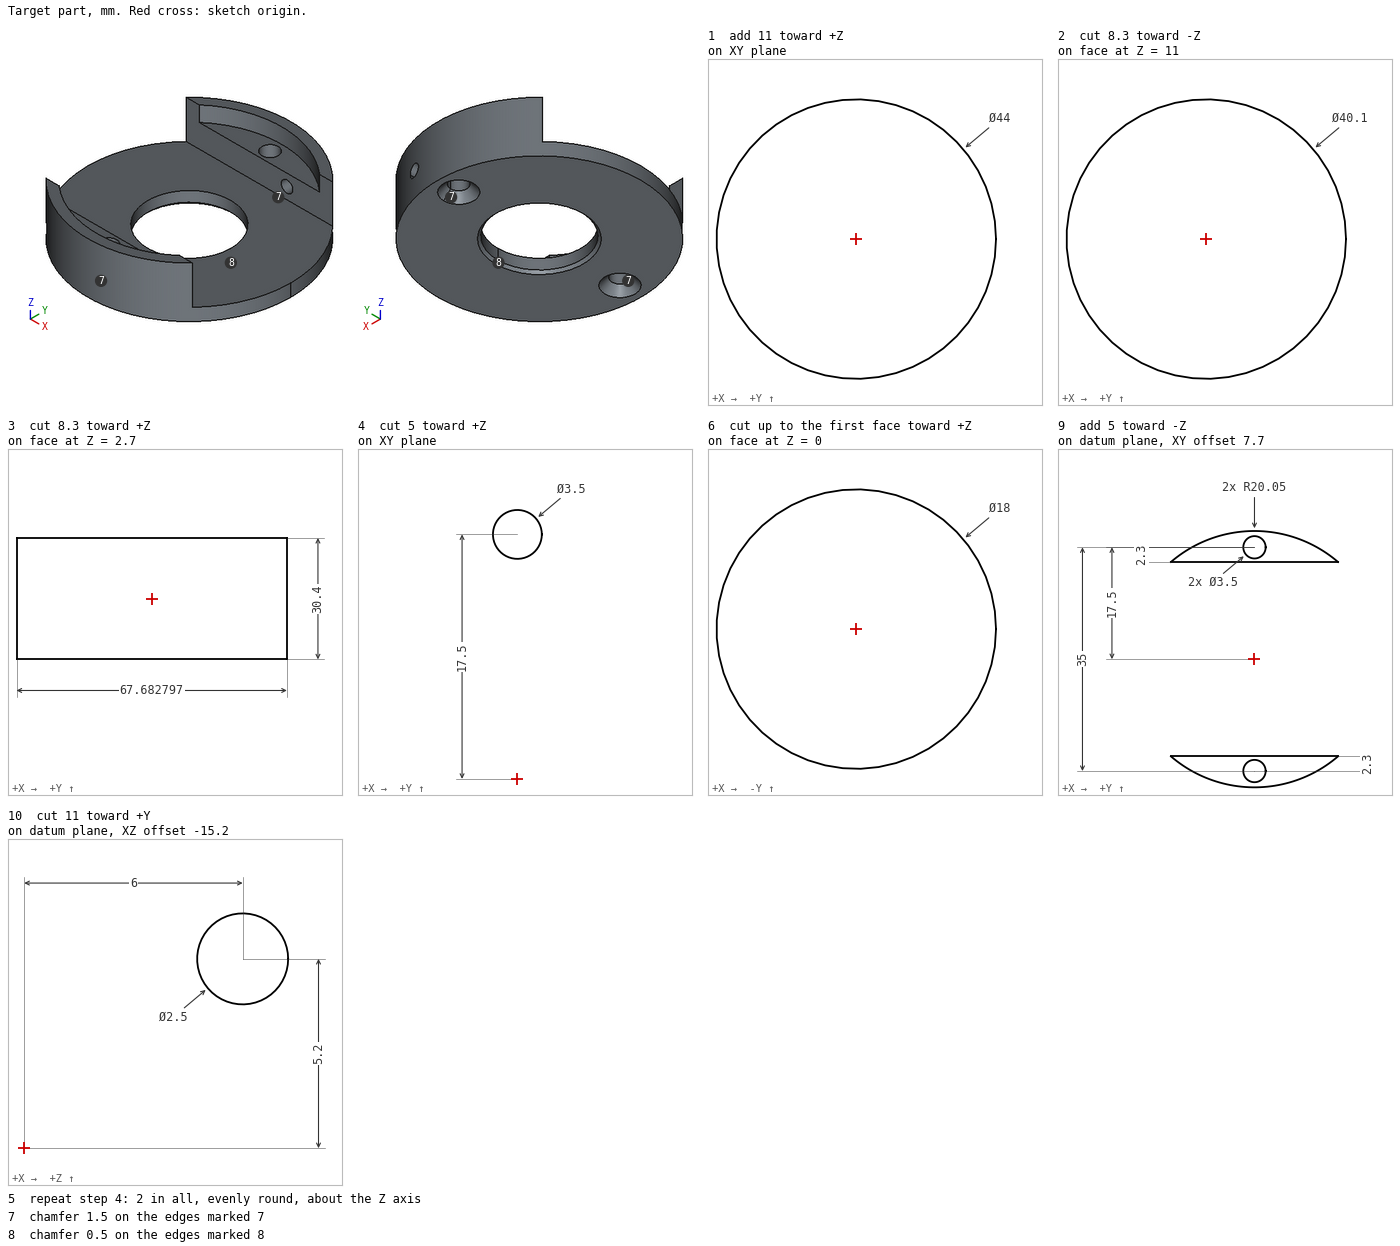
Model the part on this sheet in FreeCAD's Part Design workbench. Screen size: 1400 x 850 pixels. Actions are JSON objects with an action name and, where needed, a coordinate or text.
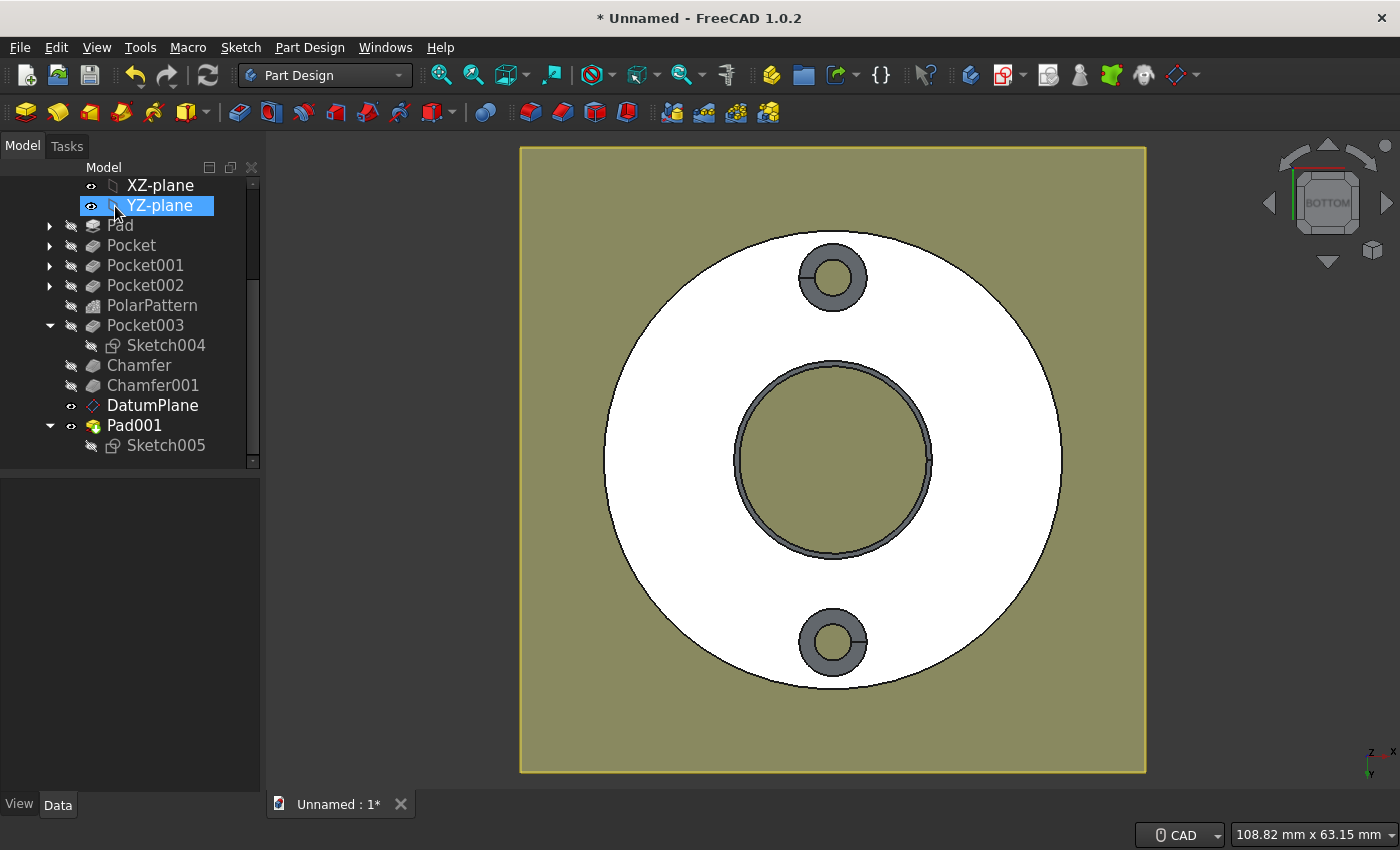
{"action": "left_click", "coordinate": [116, 406]}
{"action": "key", "text": "space"}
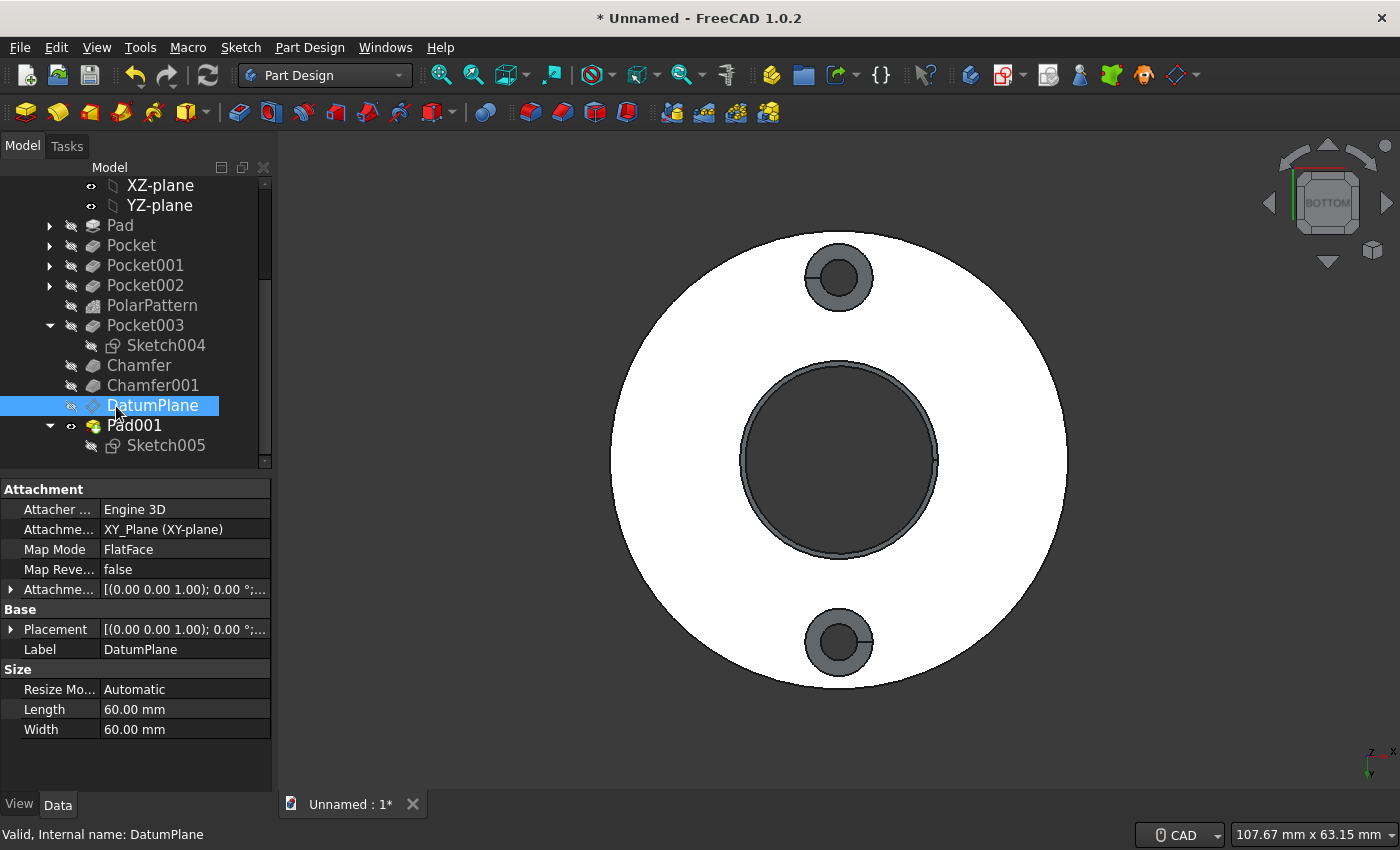
{"action": "scroll", "coordinate": [160, 321], "scroll_direction": "down", "scroll_amount": 3}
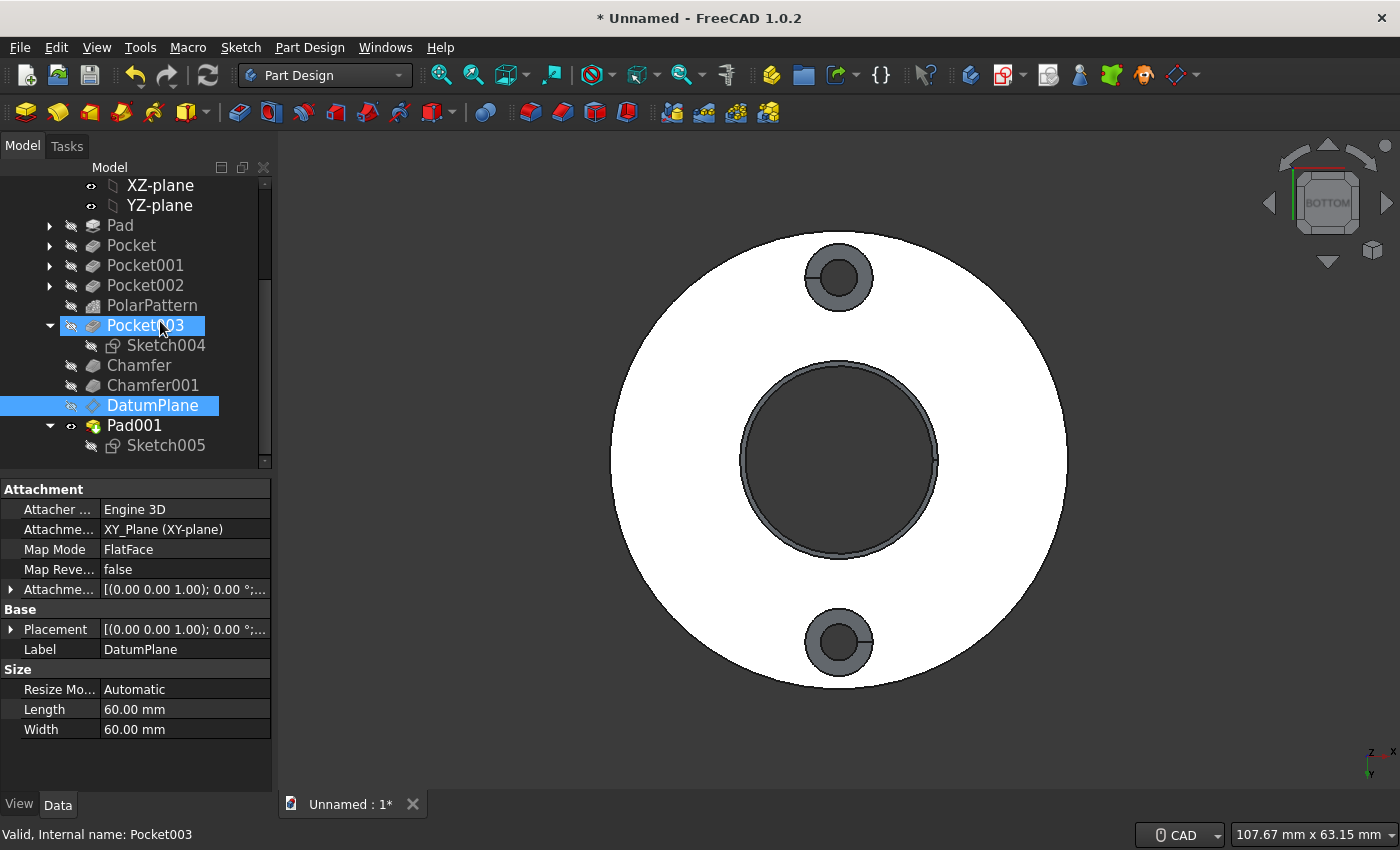
{"action": "scroll", "coordinate": [160, 321], "scroll_direction": "up", "scroll_amount": 15}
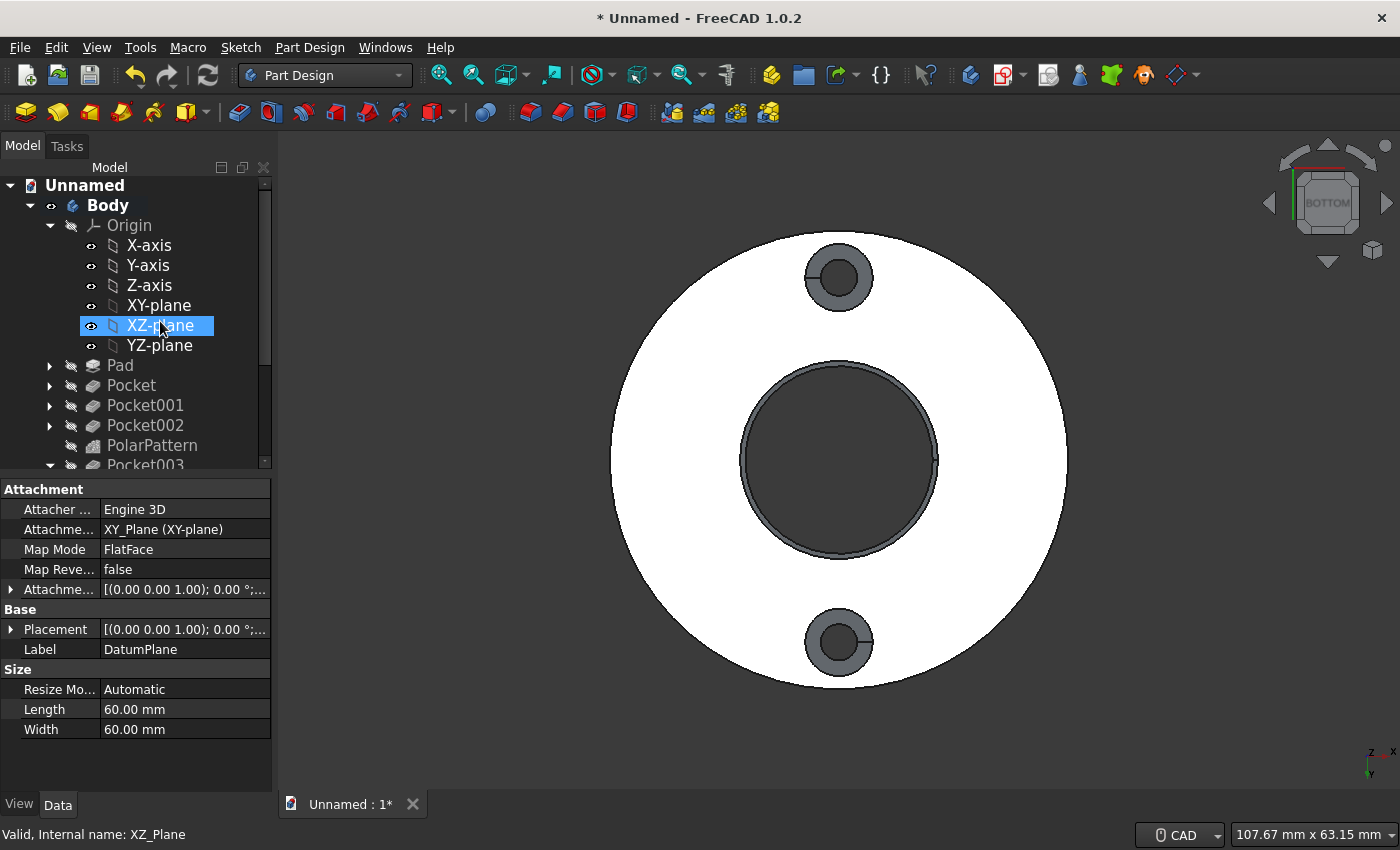
{"action": "left_click", "coordinate": [136, 326]}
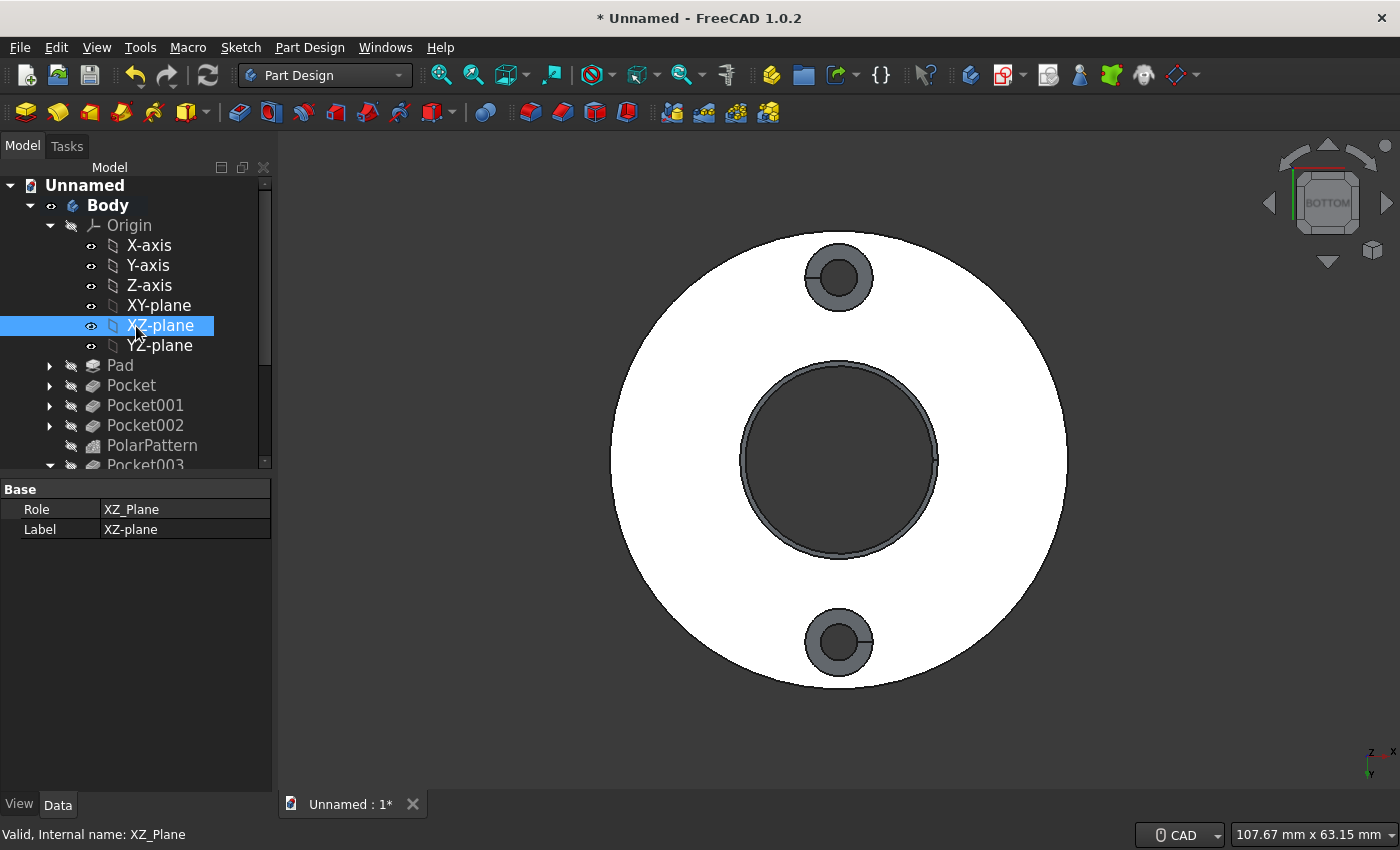
{"action": "left_click", "coordinate": [1176, 76]}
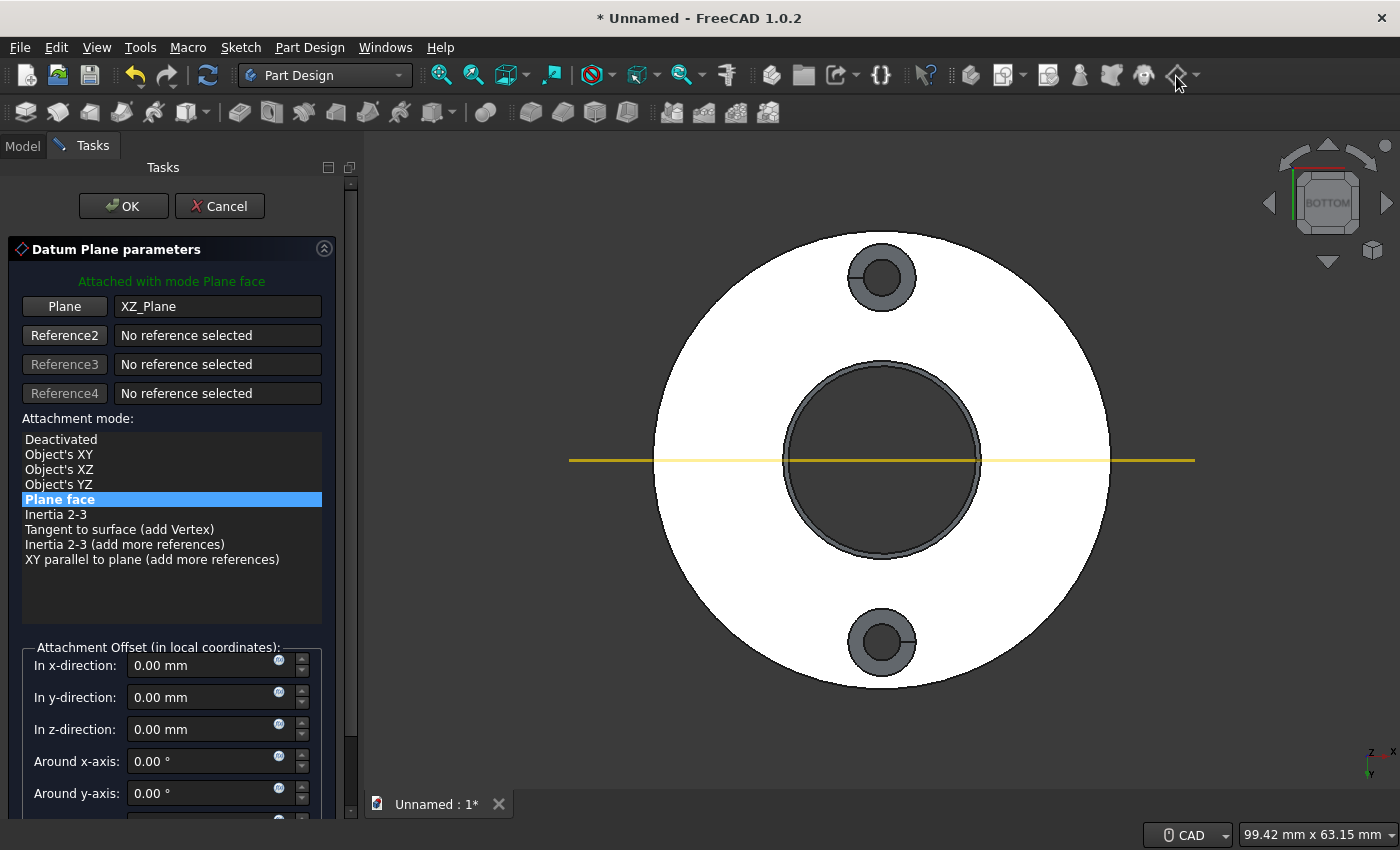
{"action": "triple_click", "coordinate": [210, 729]}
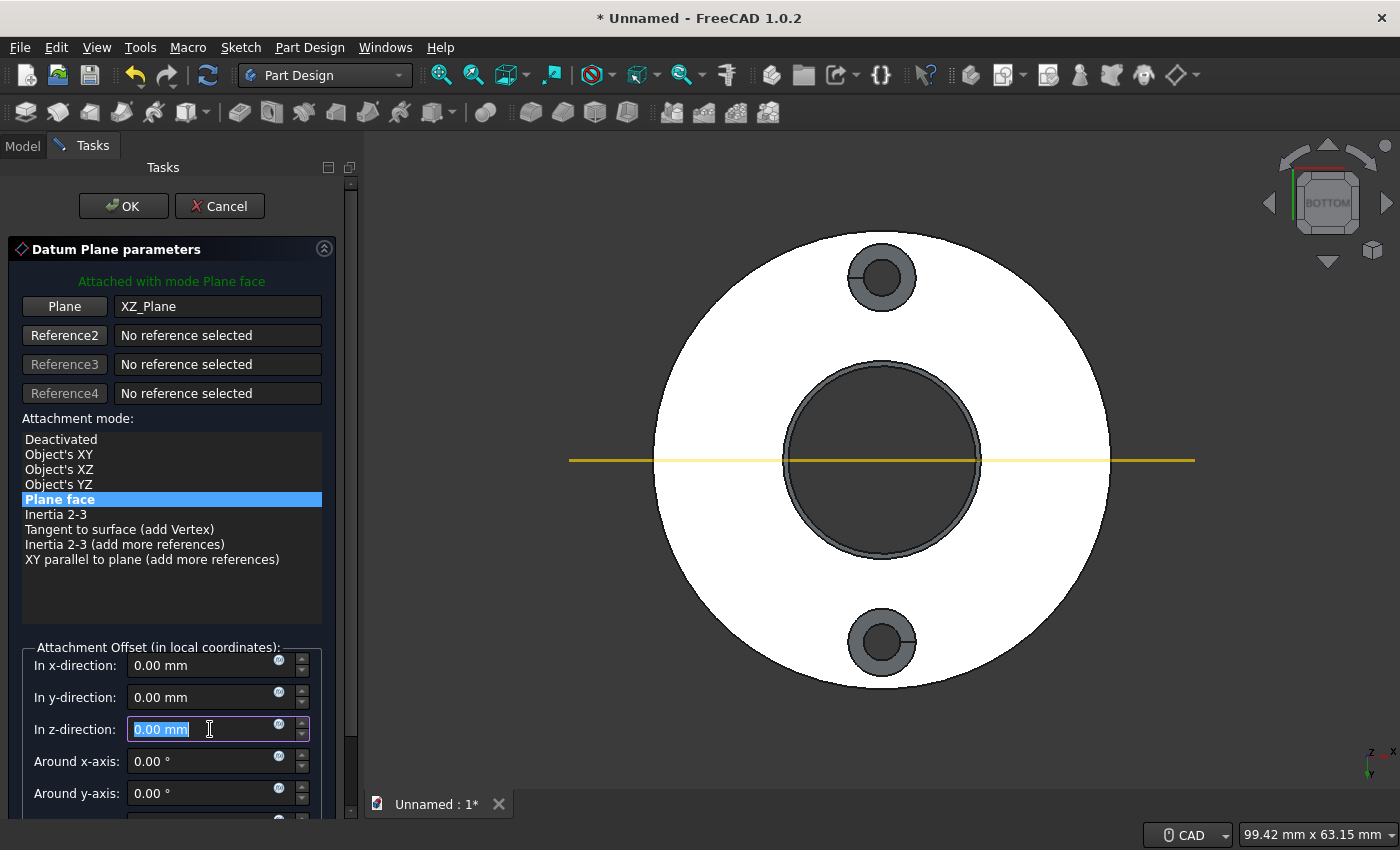
{"action": "type", "text": "-15.2"}
{"action": "key", "text": "Tab"}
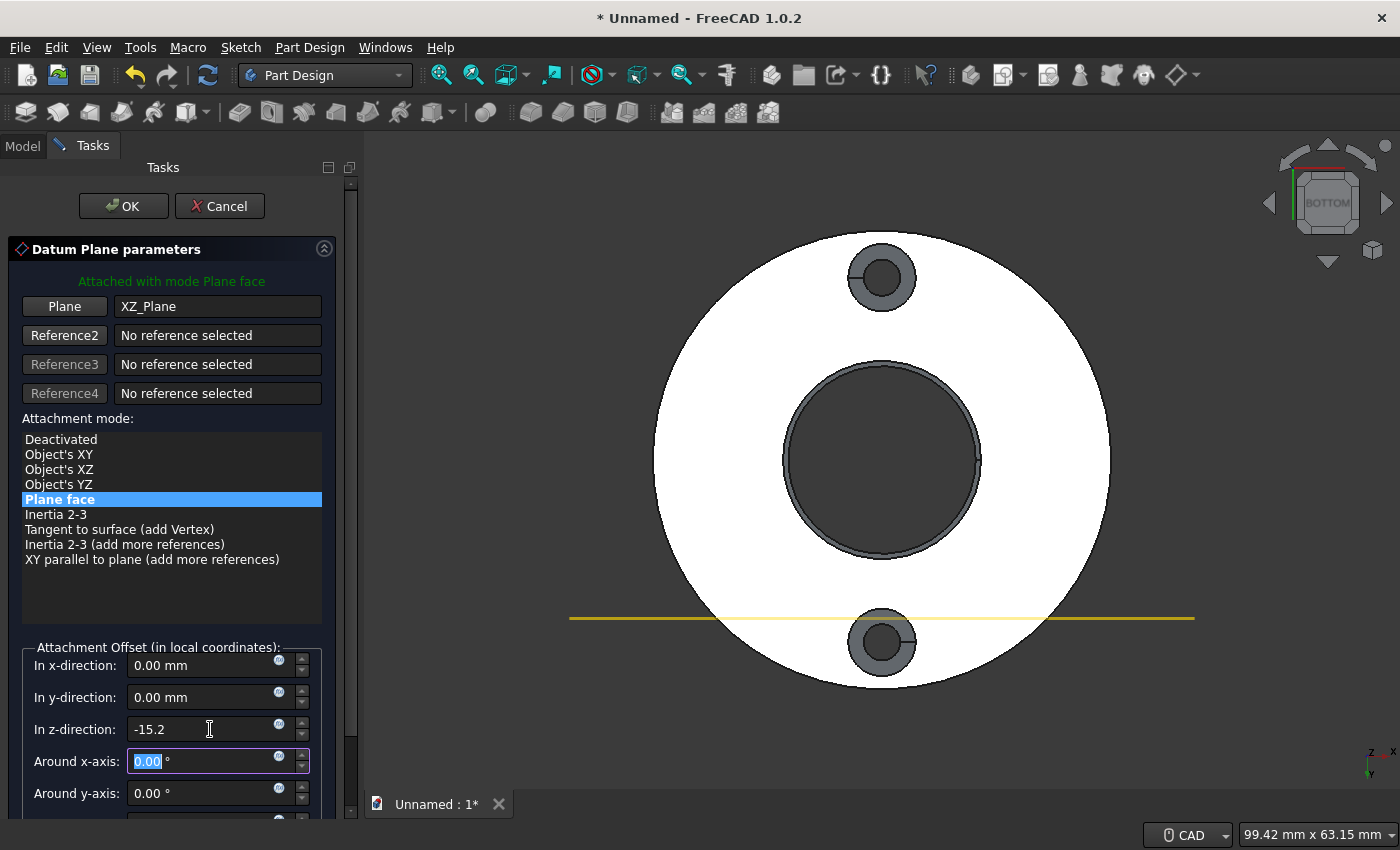
{"action": "left_click", "coordinate": [124, 206]}